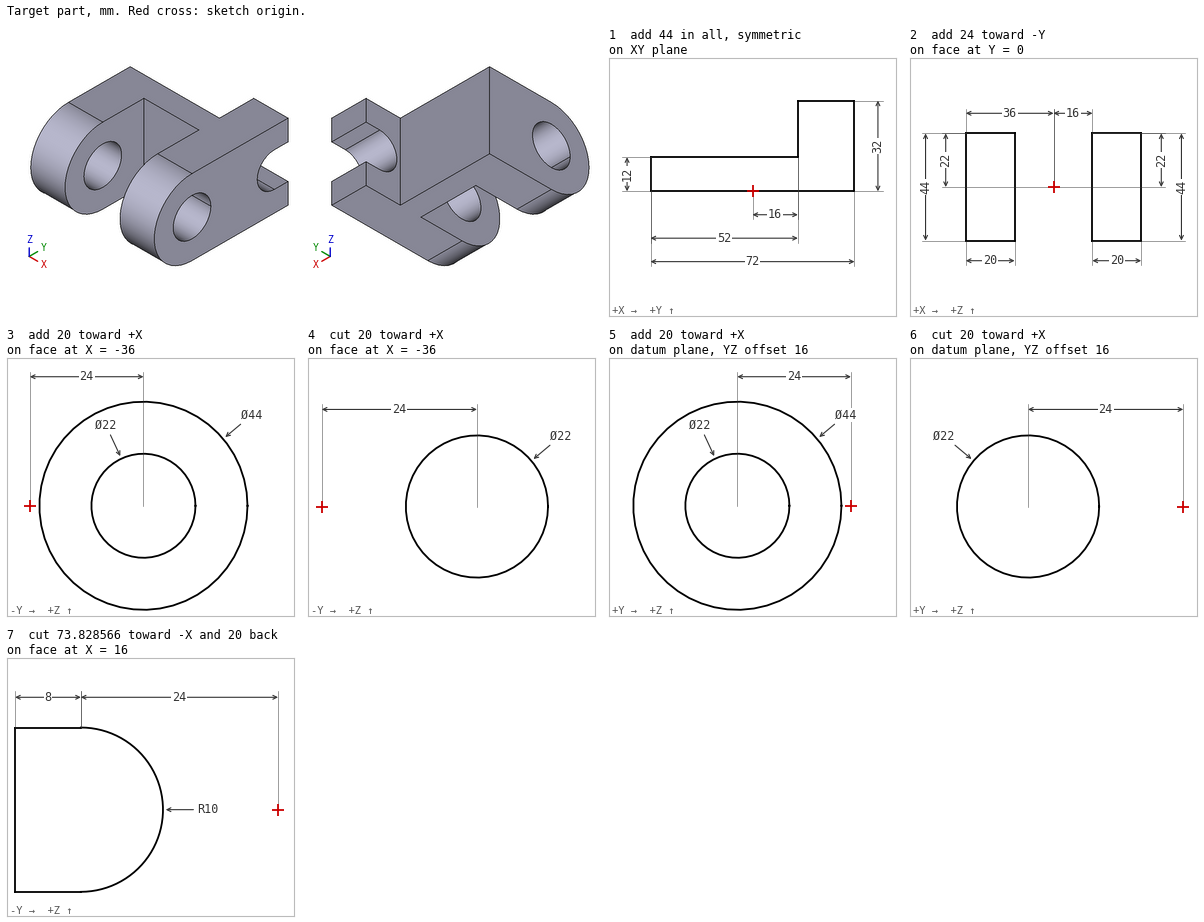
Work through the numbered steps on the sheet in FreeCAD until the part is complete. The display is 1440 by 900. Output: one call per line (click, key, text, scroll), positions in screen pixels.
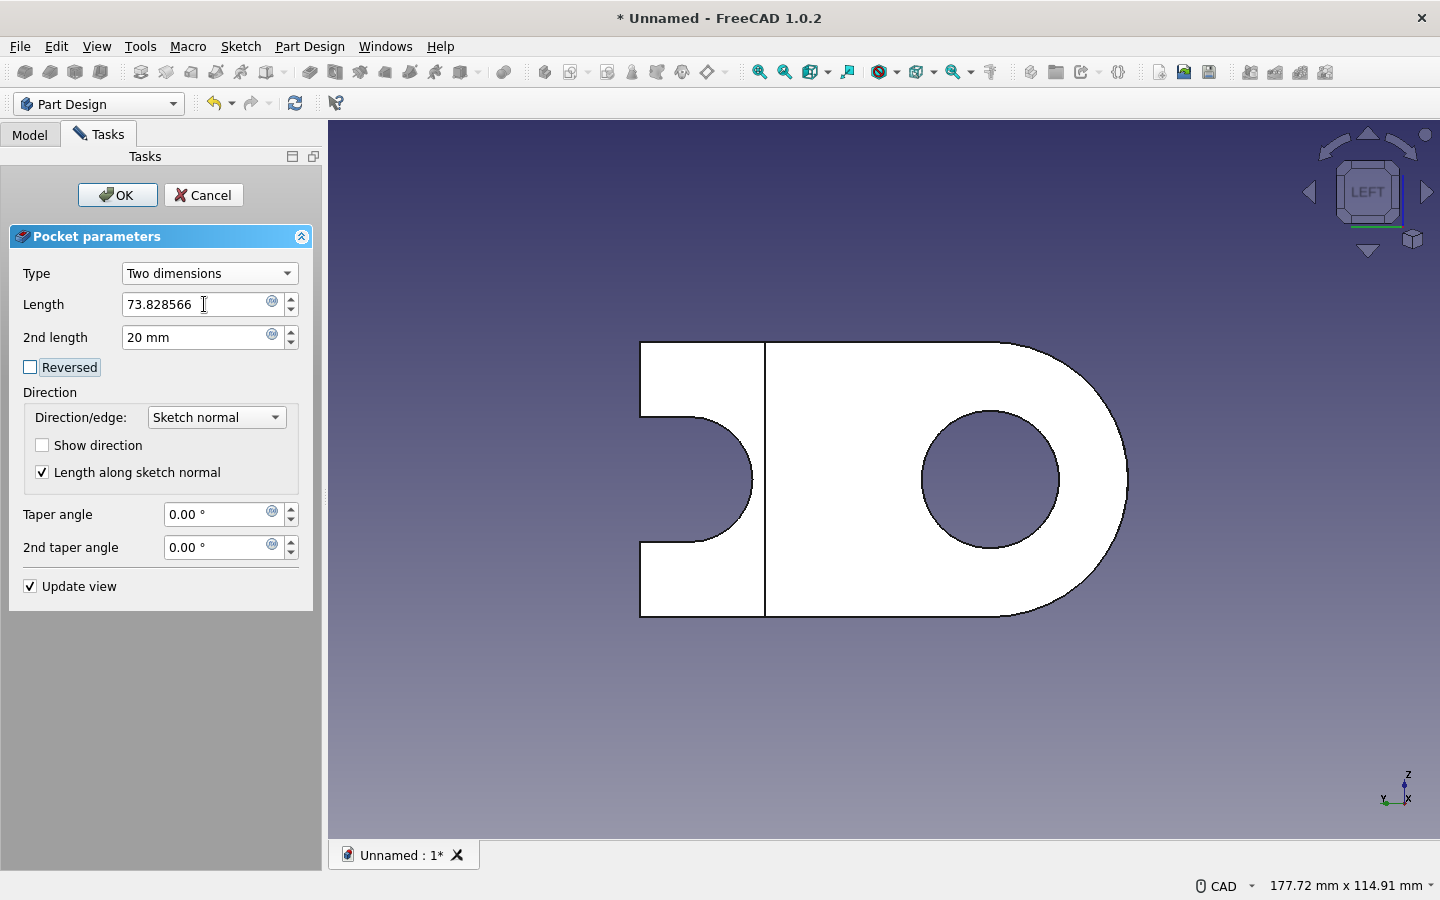
click(31, 367)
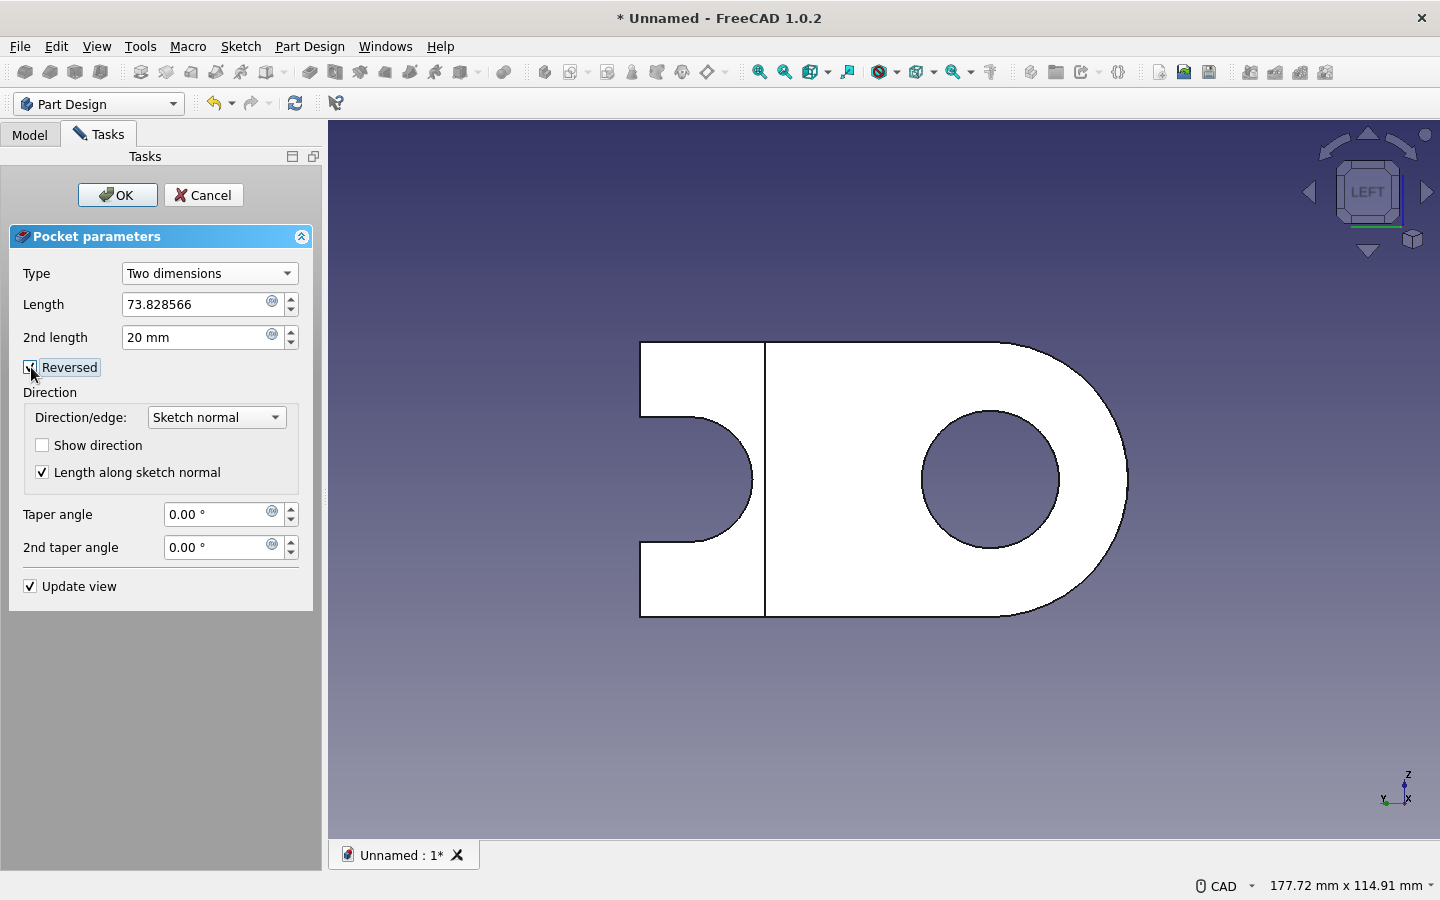
click(118, 195)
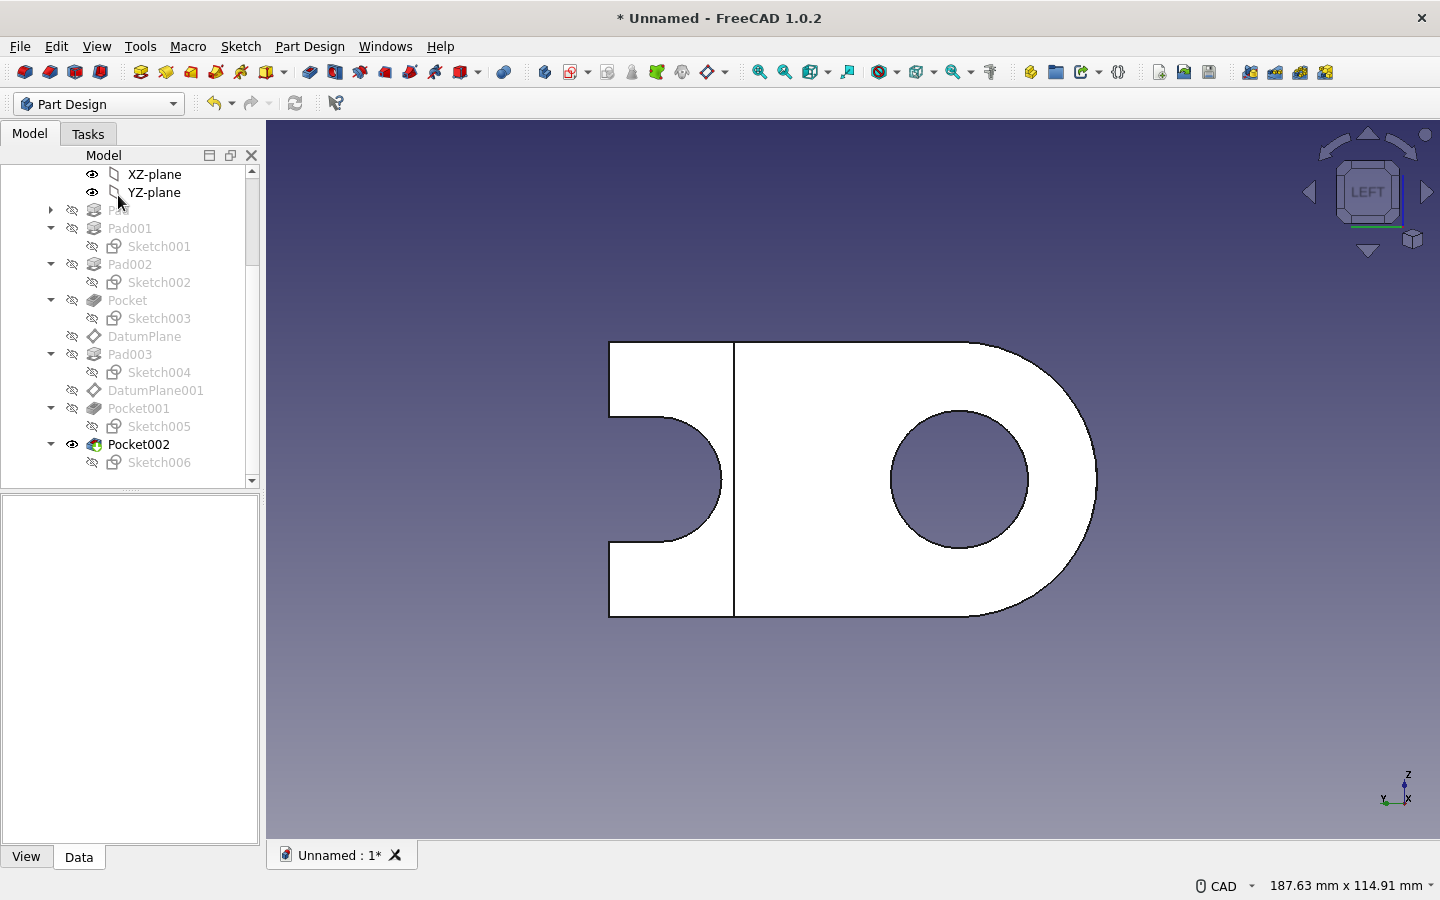
key(0)